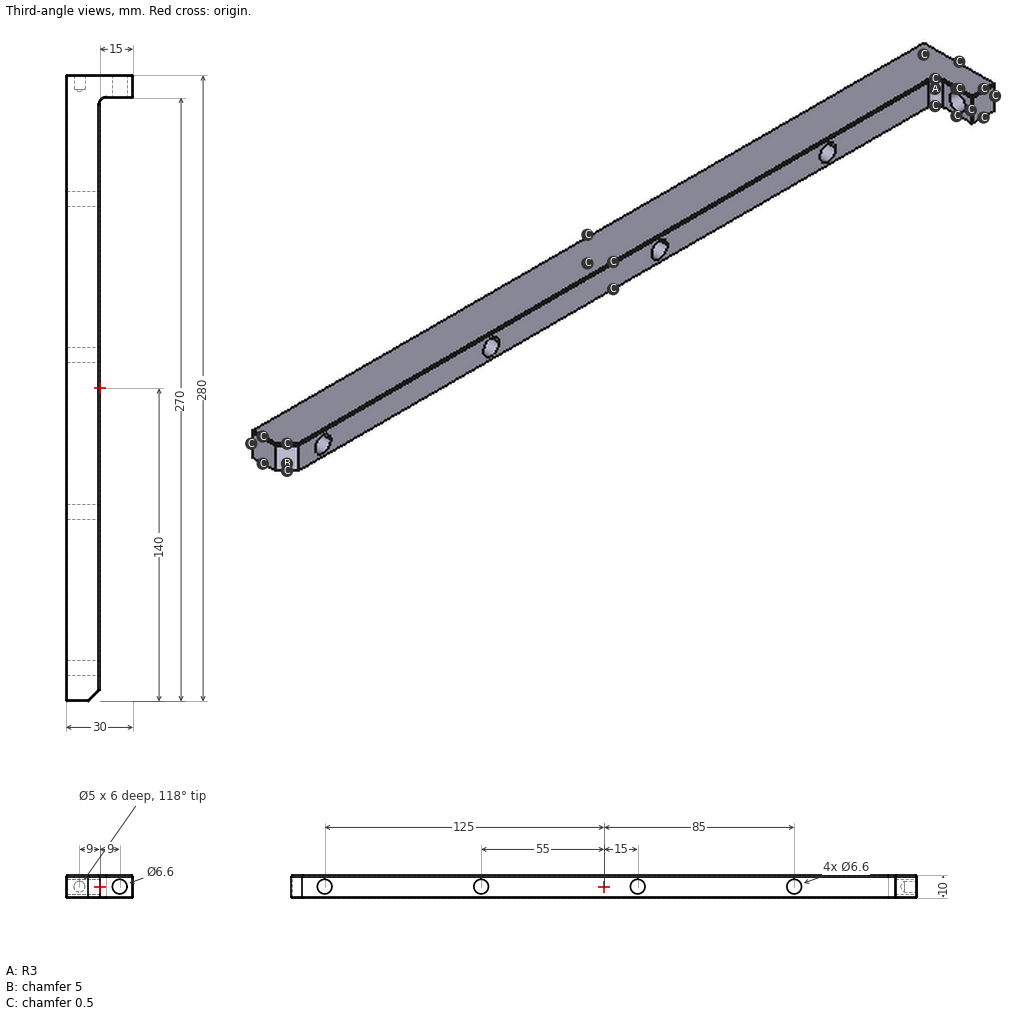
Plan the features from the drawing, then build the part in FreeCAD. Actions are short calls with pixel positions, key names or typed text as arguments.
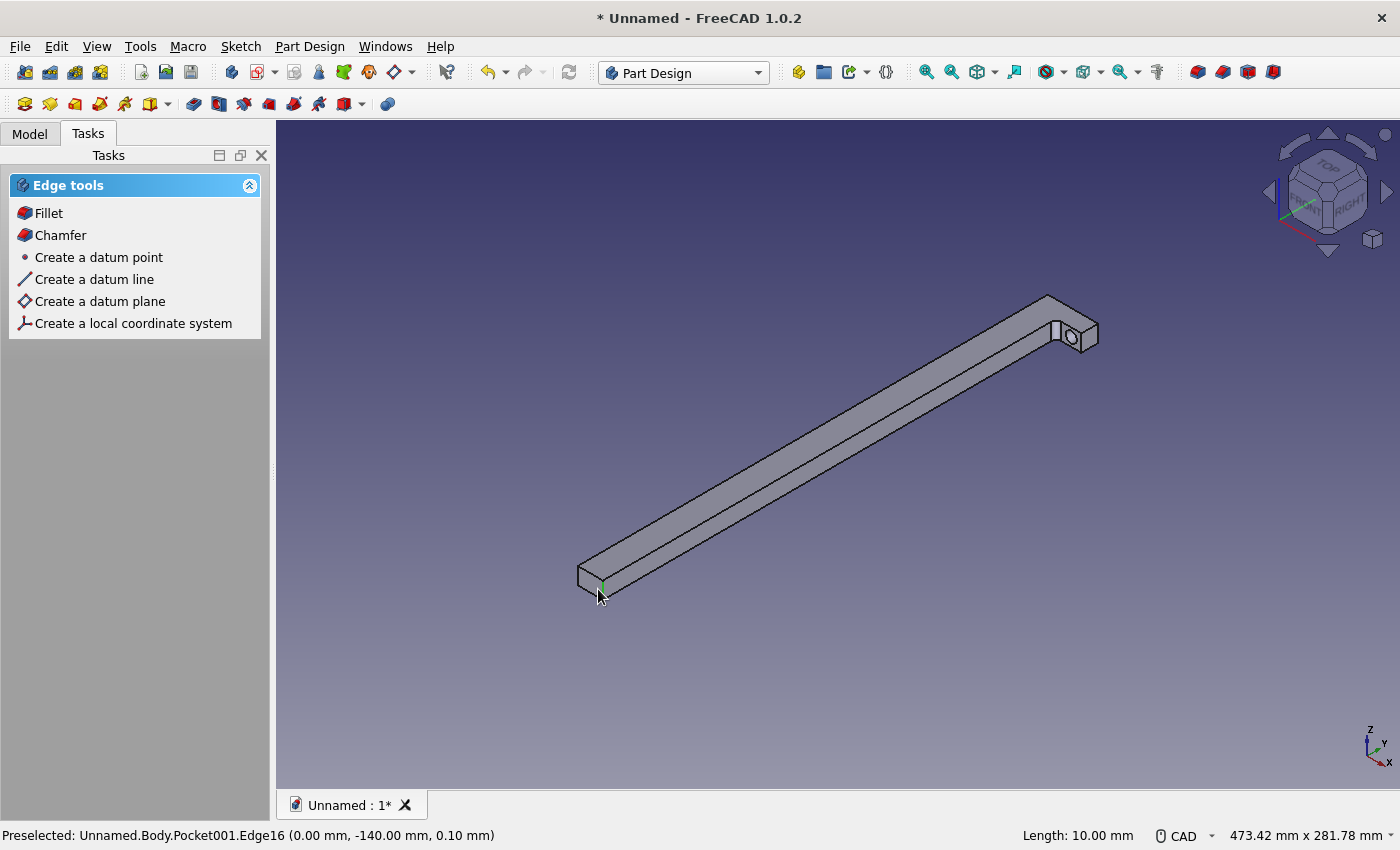
click(1223, 72)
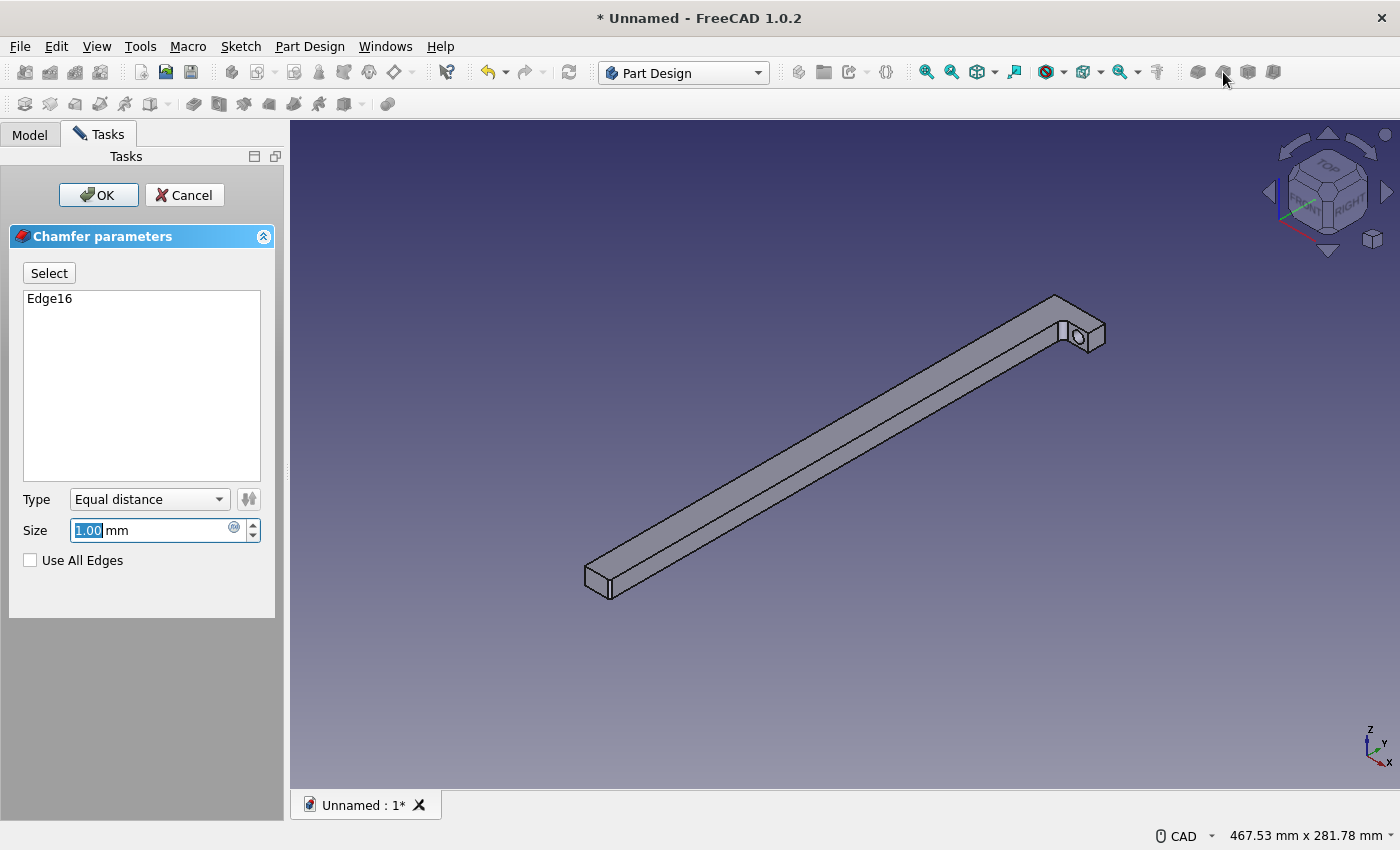
text(5)
key(Tab)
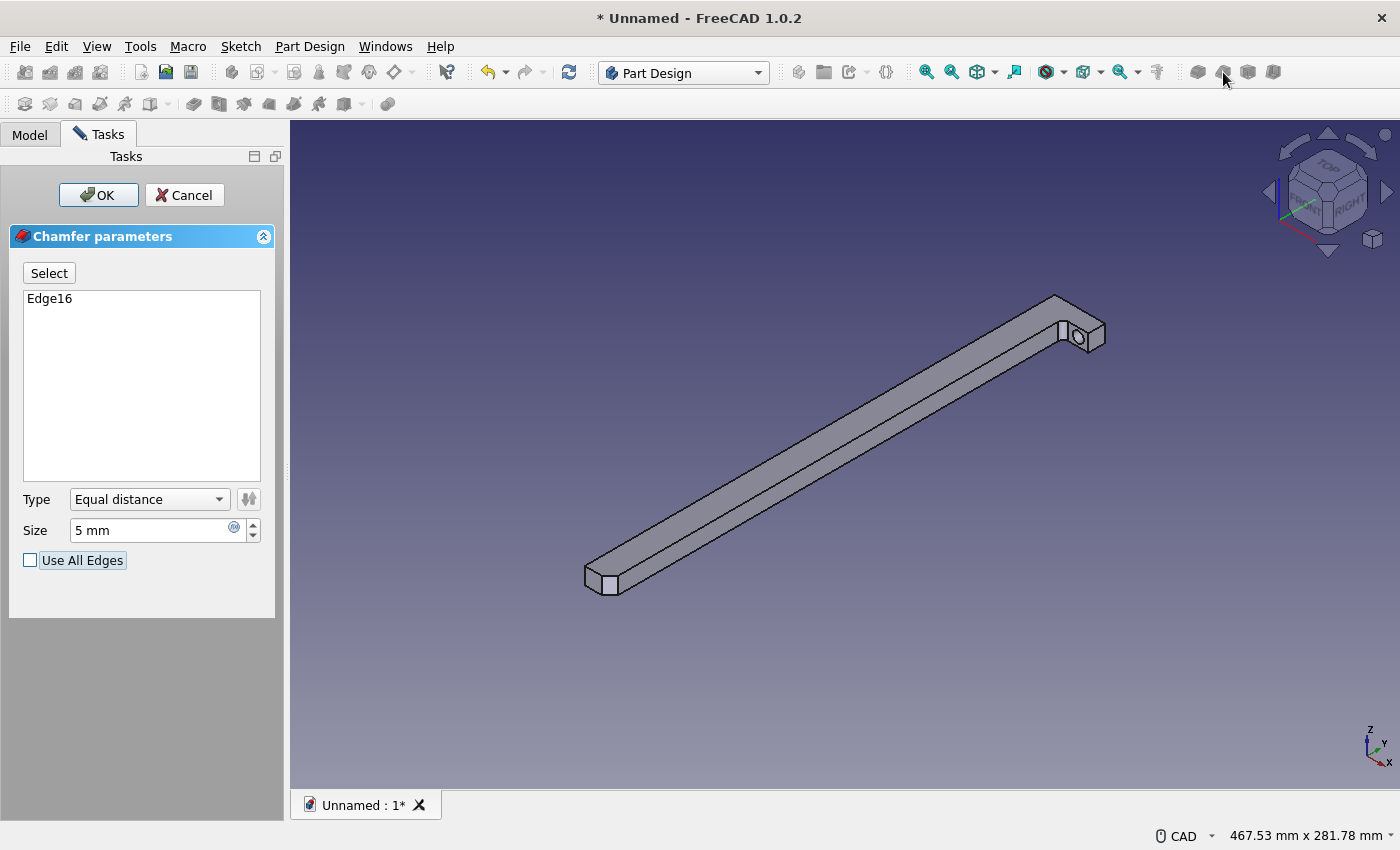
click(99, 195)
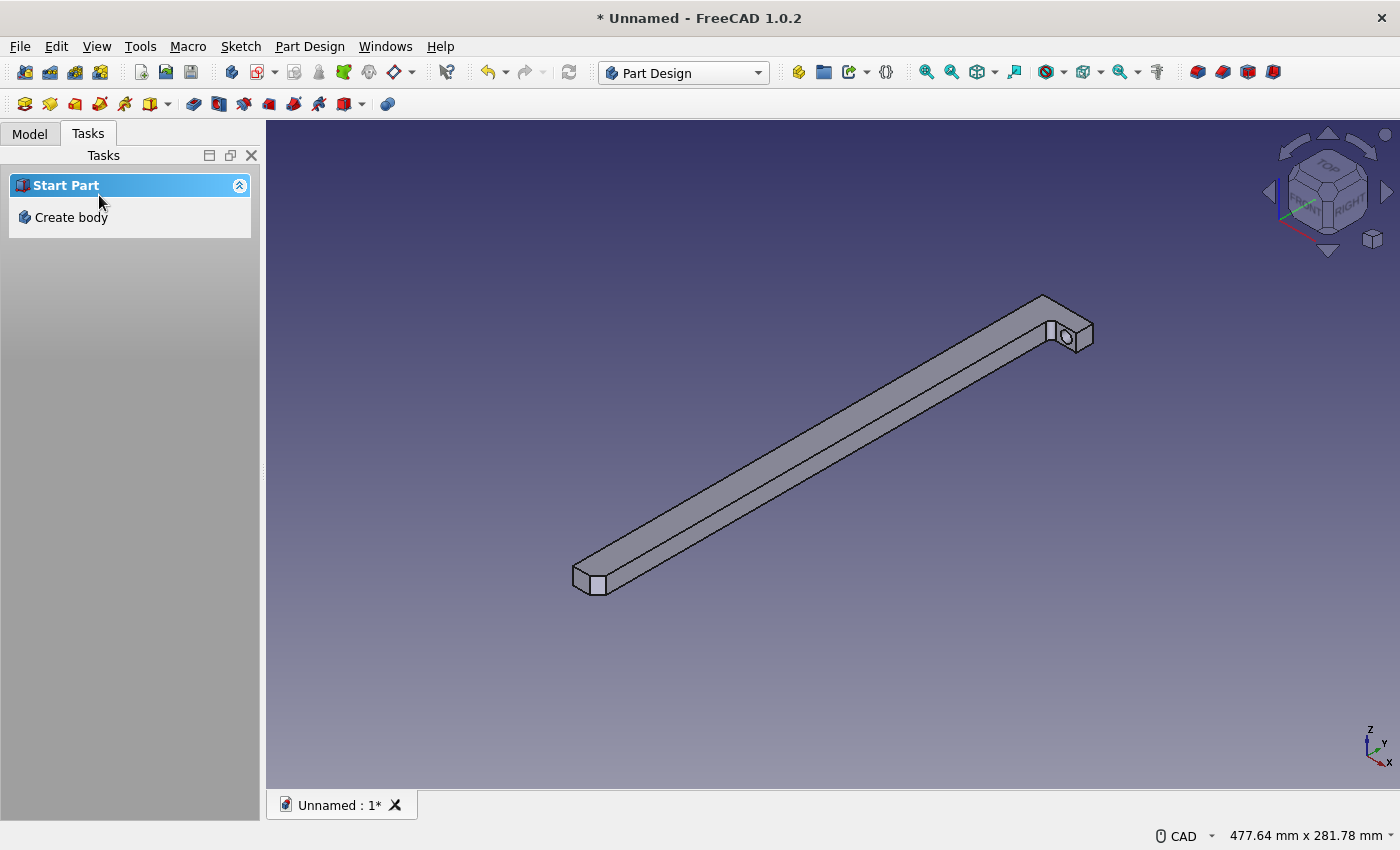
key(3)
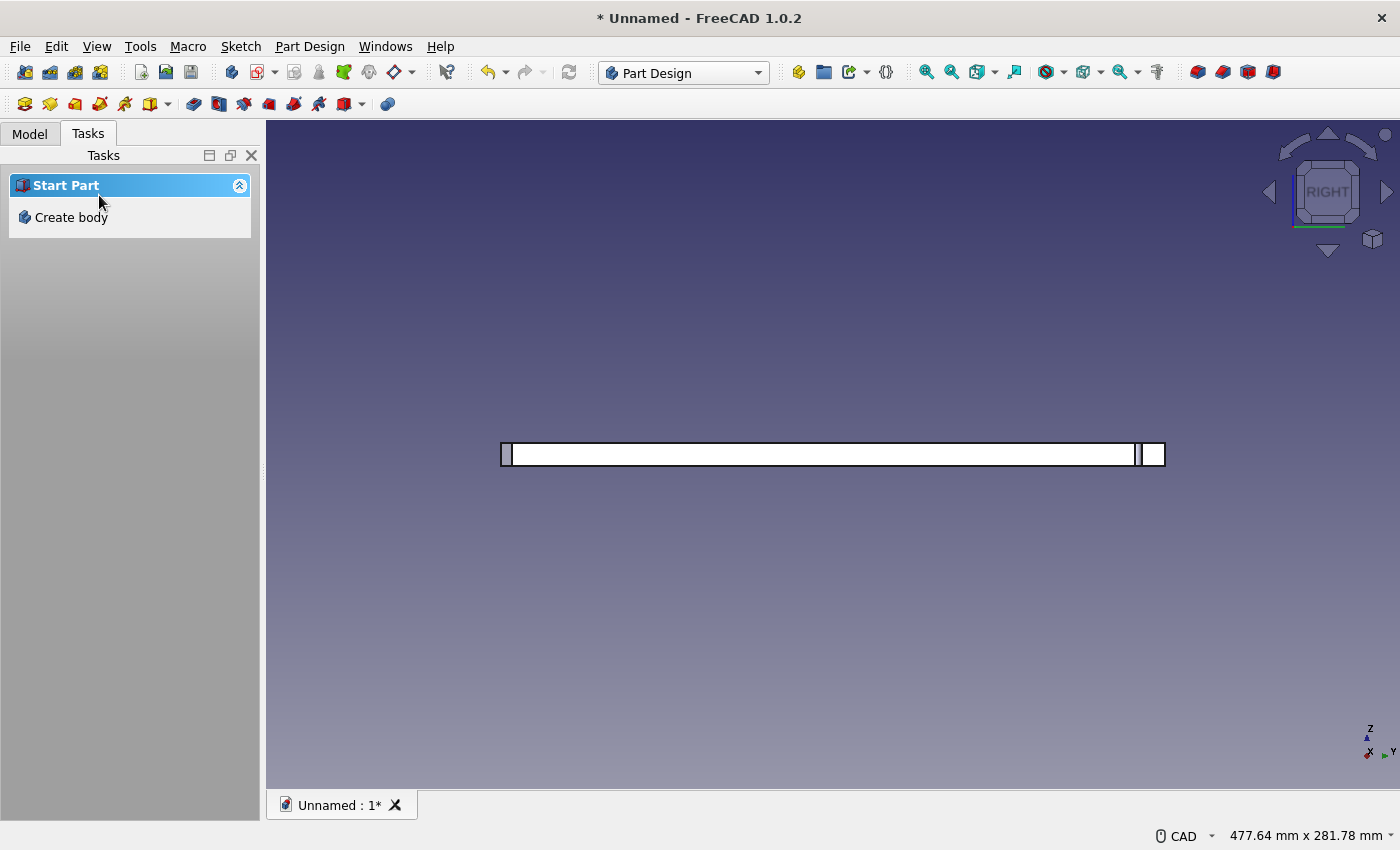
click(1090, 453)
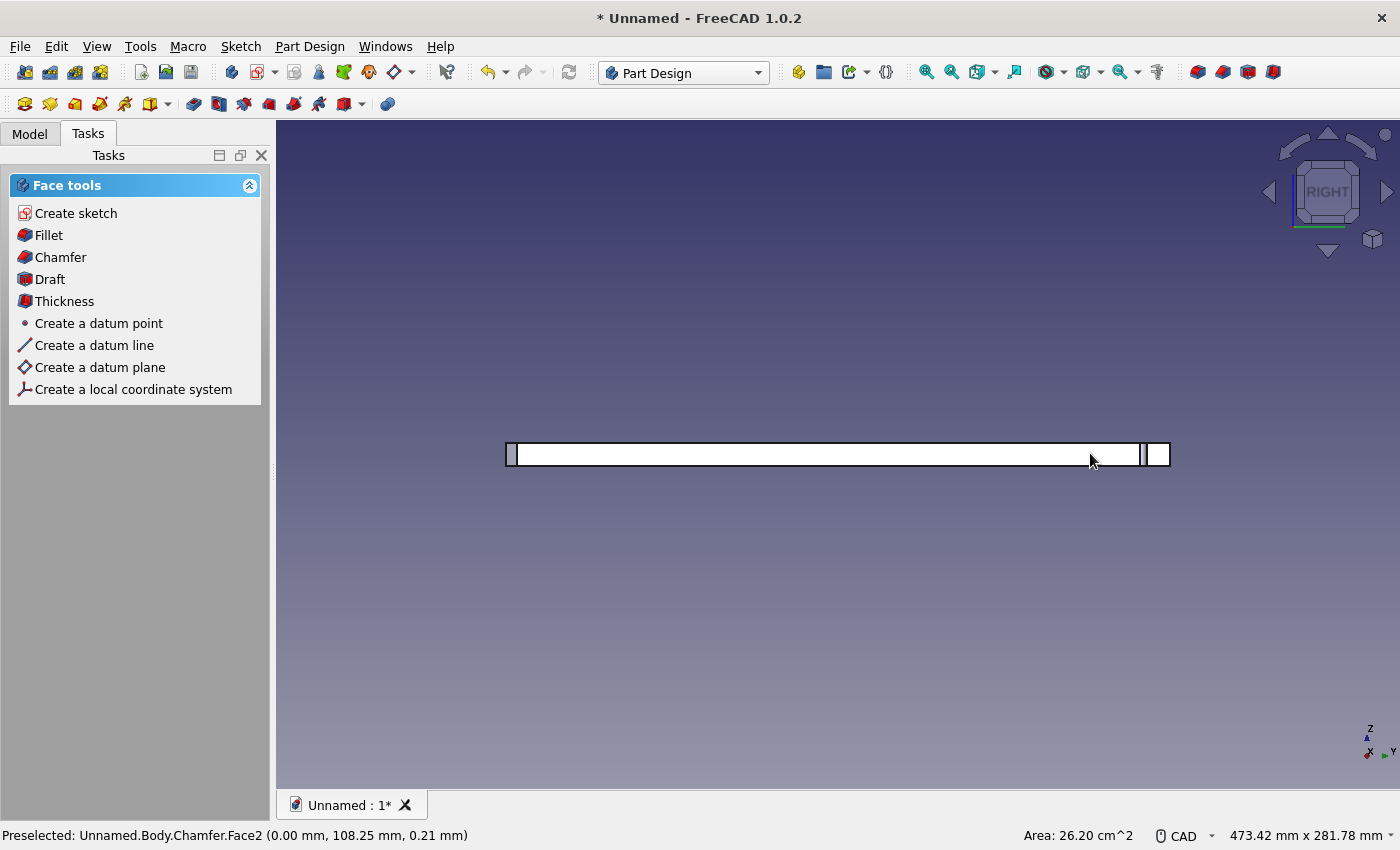
click(256, 72)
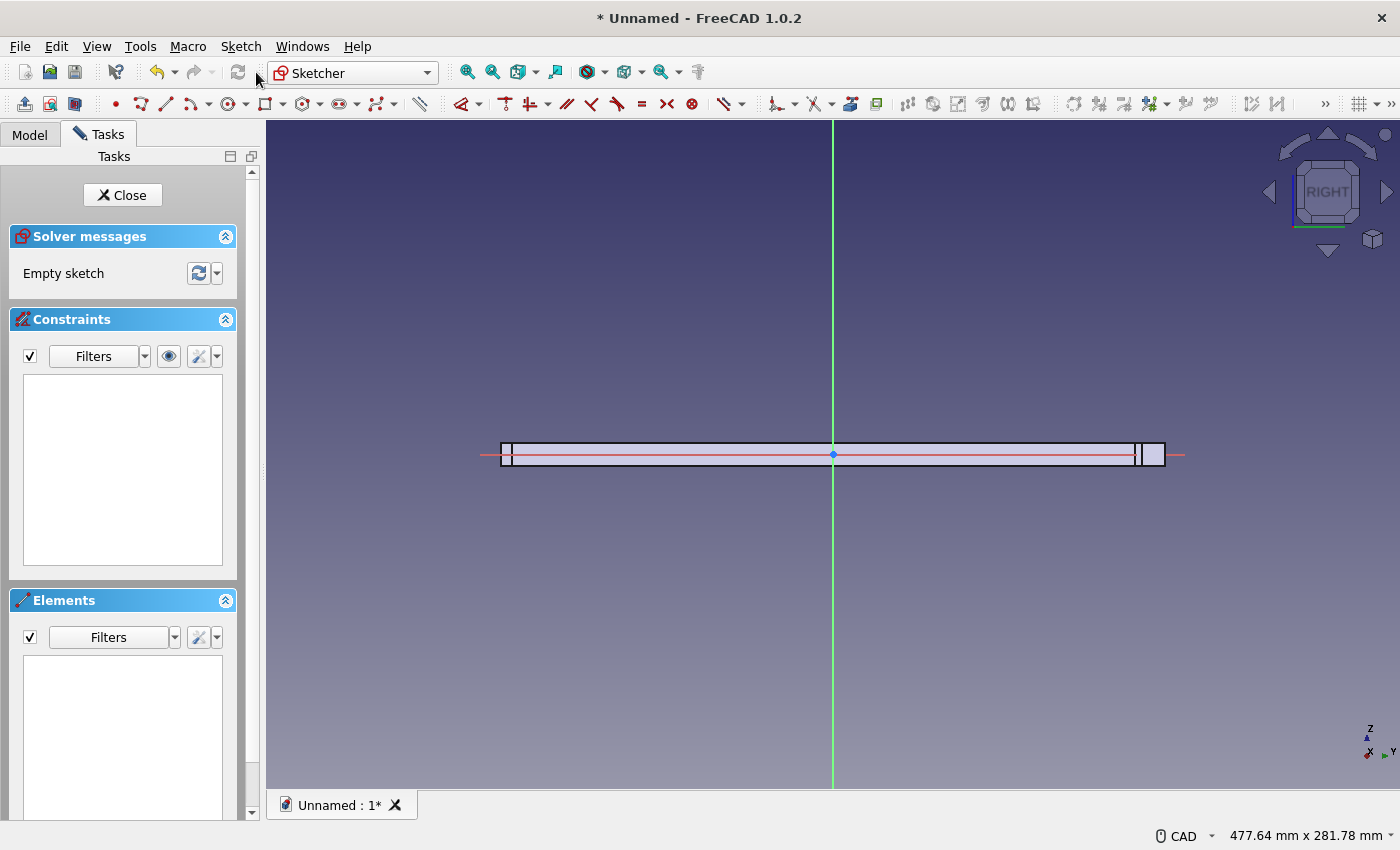
key(g)
key(c)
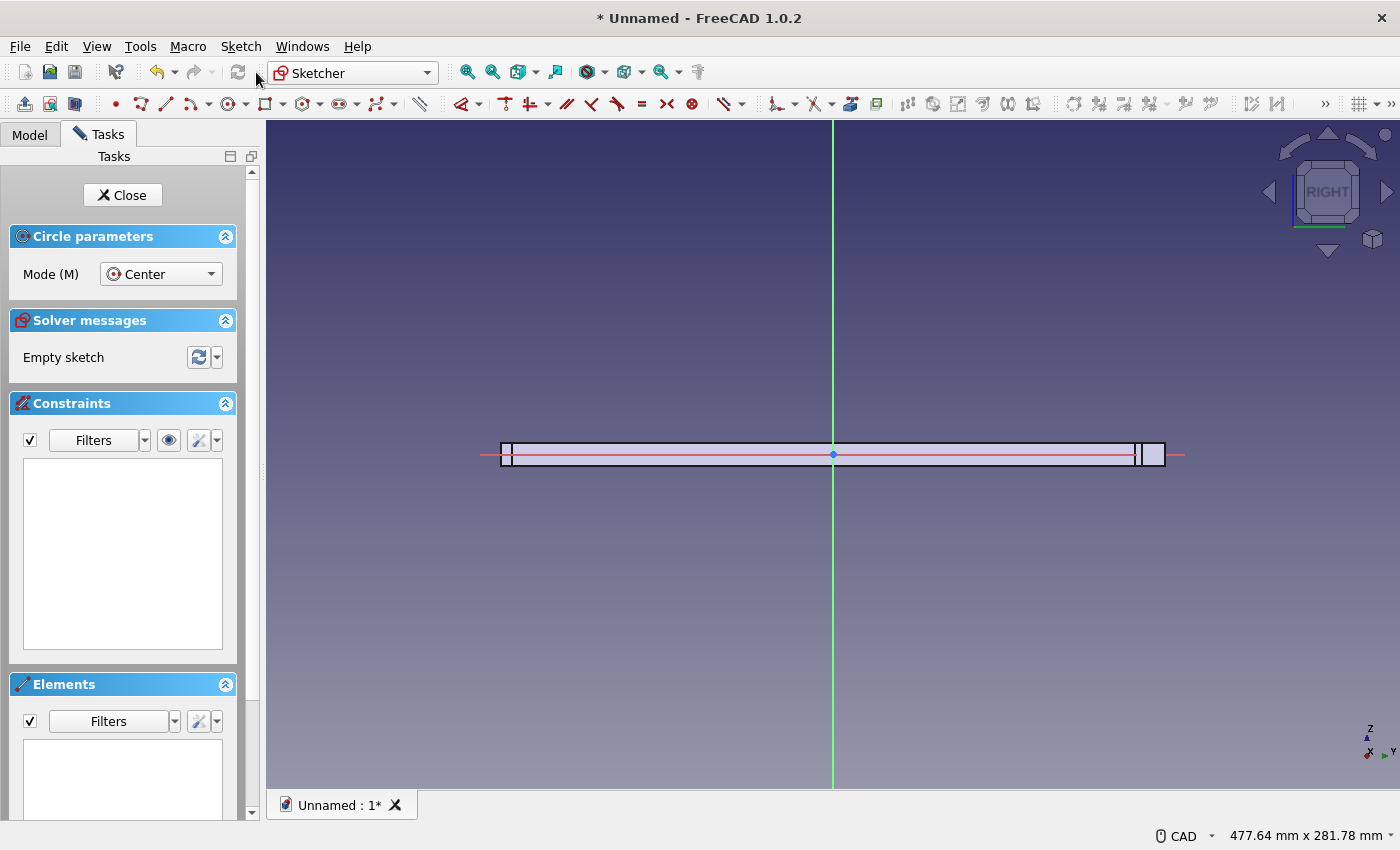
scroll(1035, 454, up, 6)